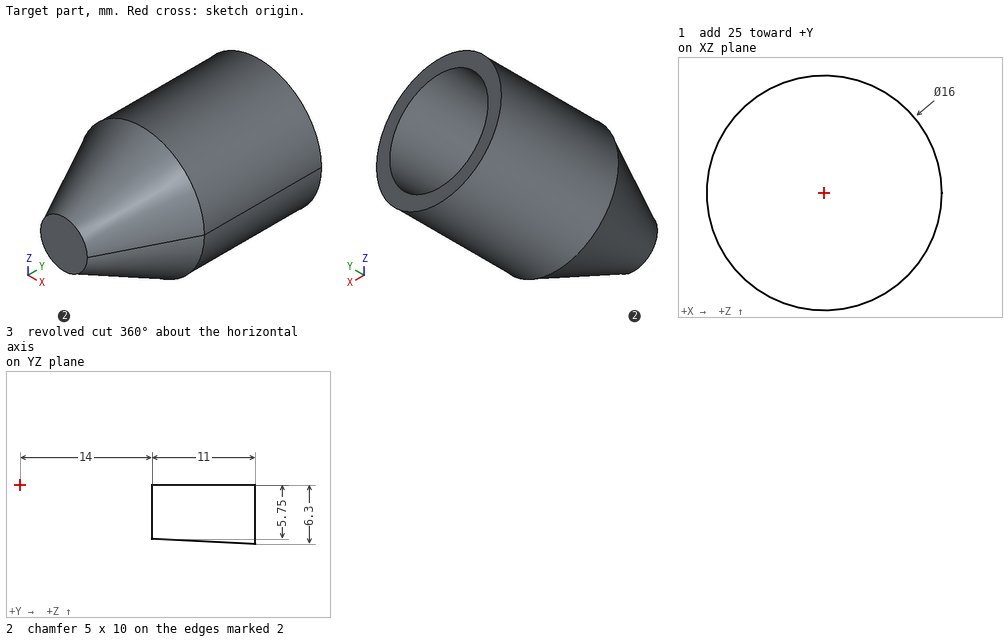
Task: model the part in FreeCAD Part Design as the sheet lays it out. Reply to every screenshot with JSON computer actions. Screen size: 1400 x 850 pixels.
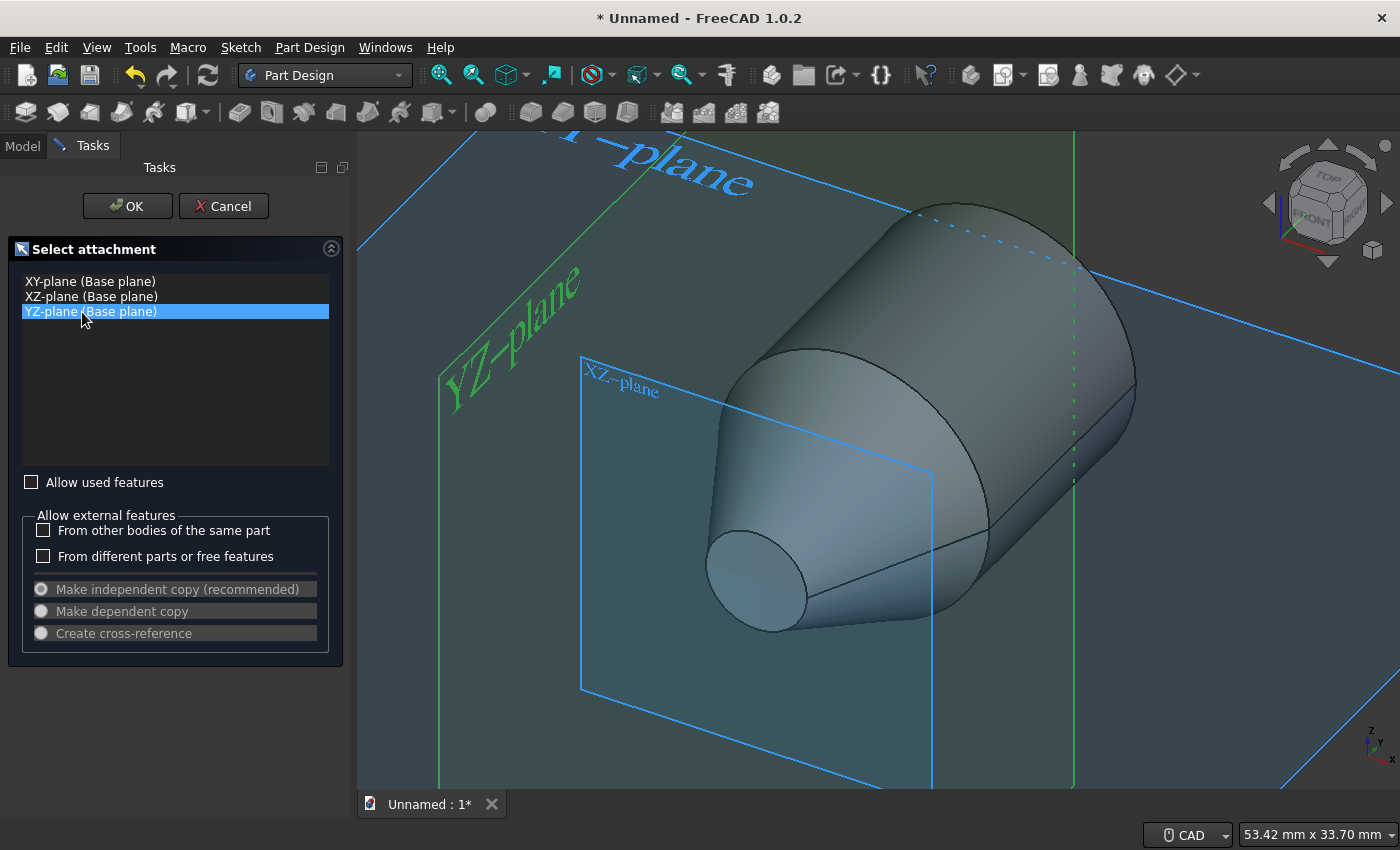
{"action": "left_click", "coordinate": [128, 206]}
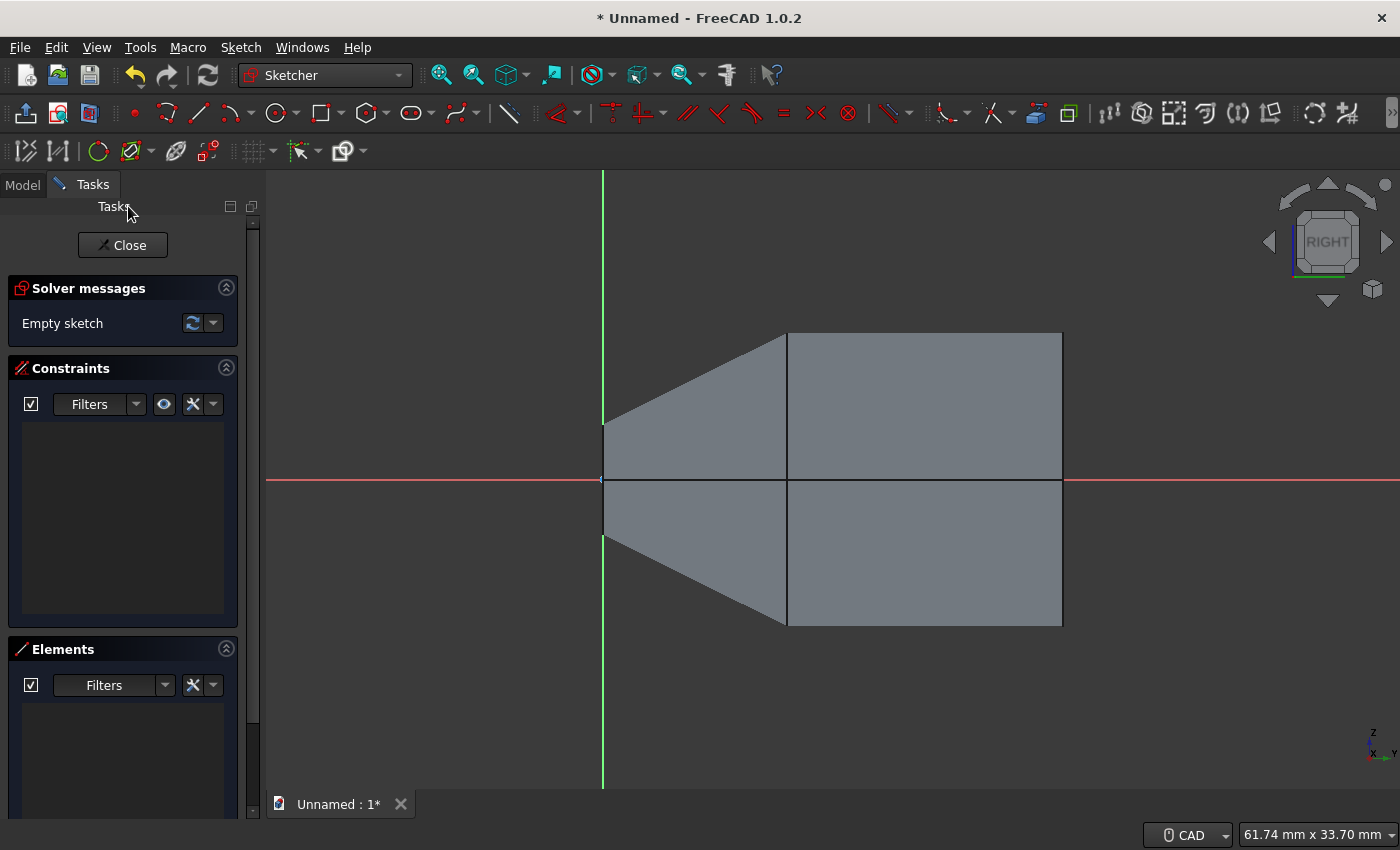
{"action": "left_click", "coordinate": [90, 114]}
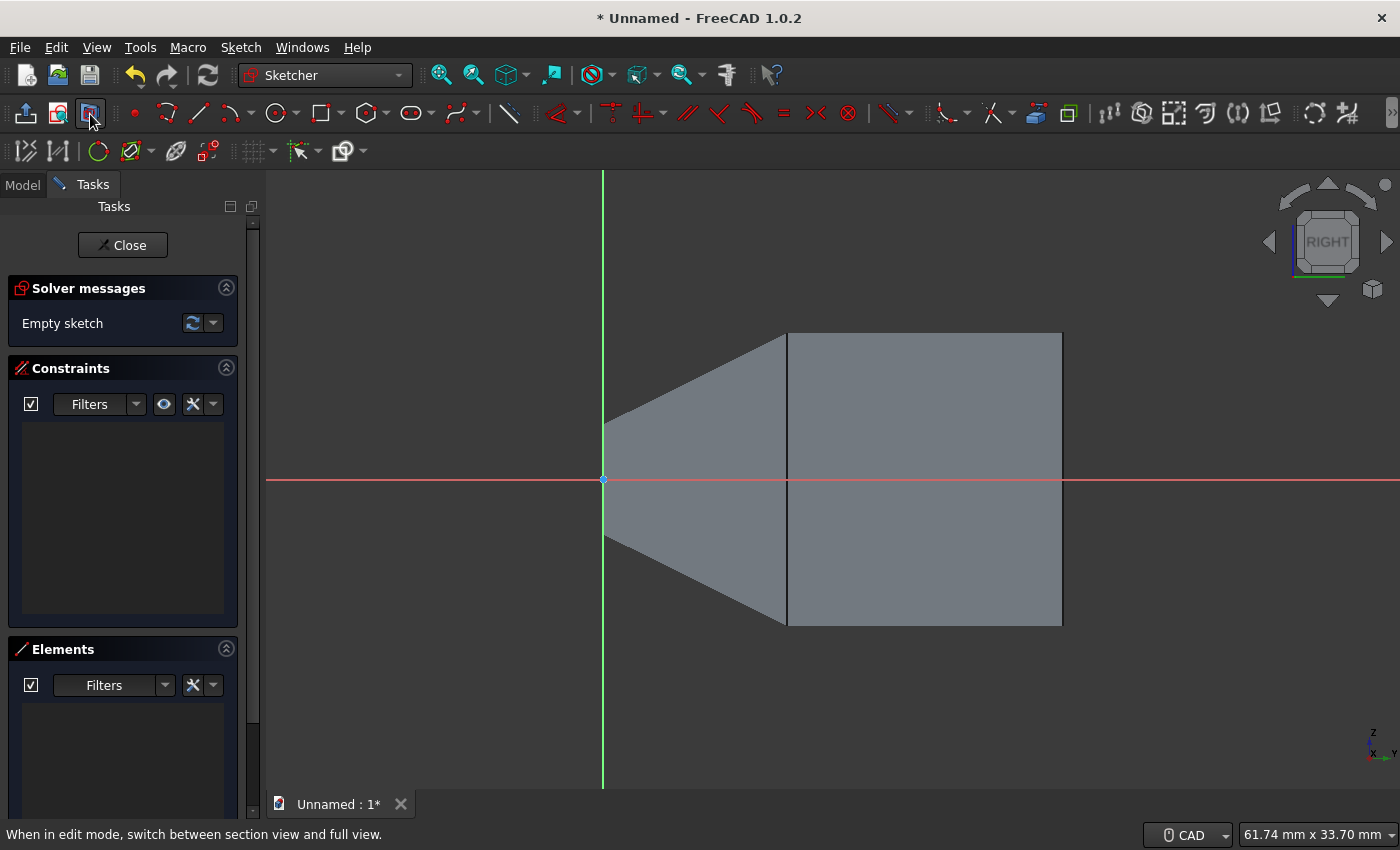
{"action": "scroll", "coordinate": [972, 655], "scroll_direction": "up", "scroll_amount": 2}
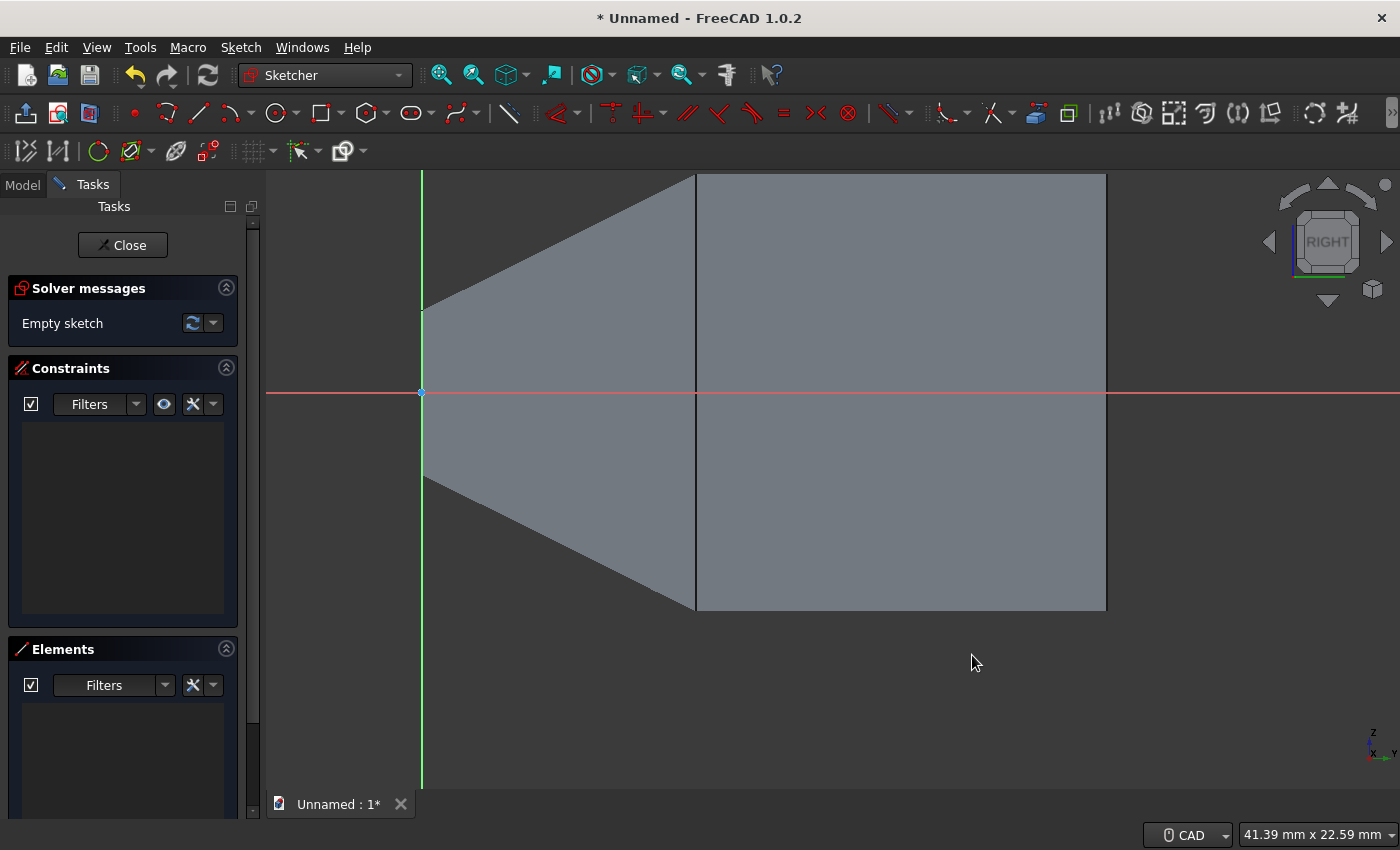
{"action": "left_click", "coordinate": [168, 114]}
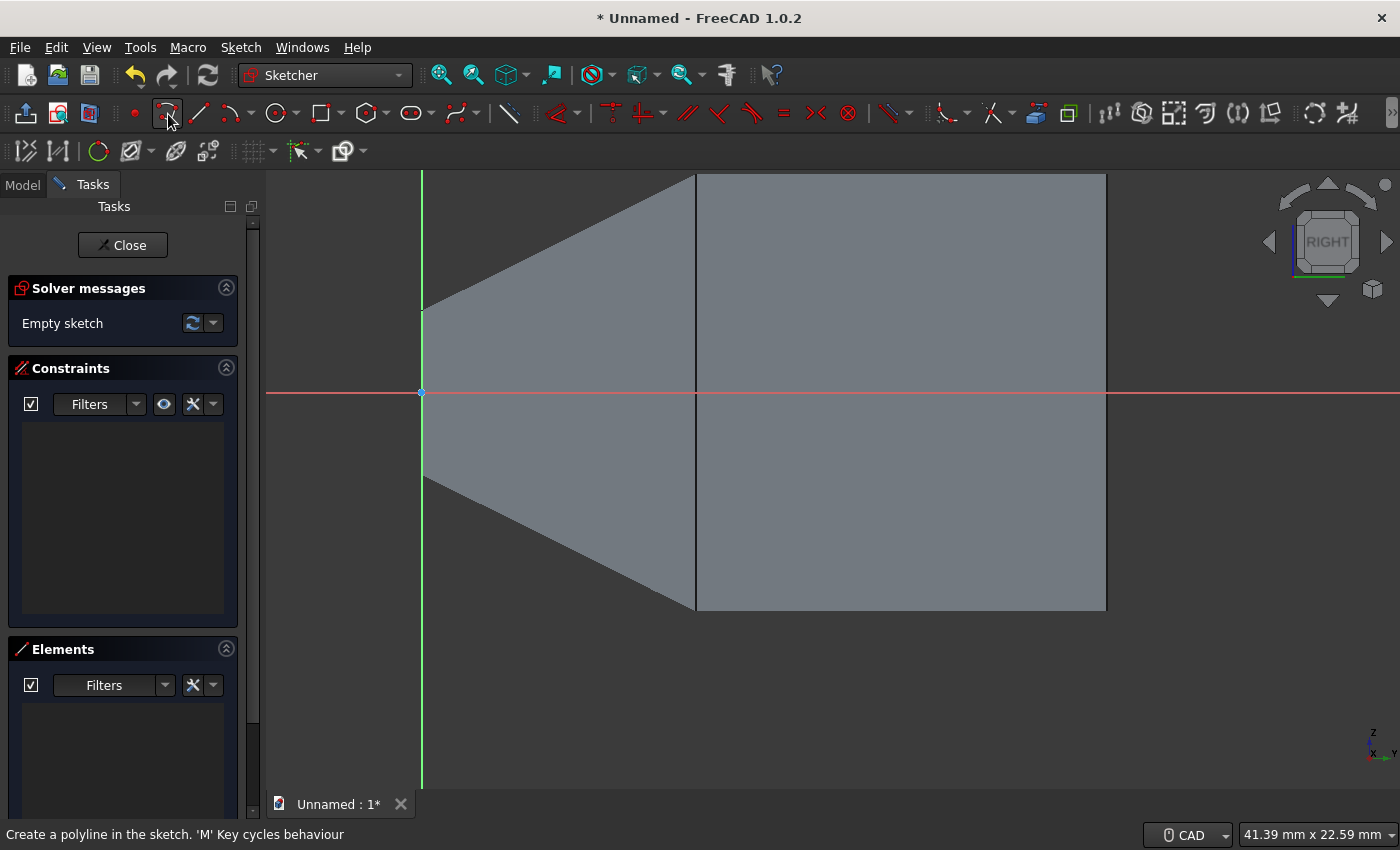
{"action": "left_click", "coordinate": [805, 393]}
{"action": "left_click", "coordinate": [805, 550]}
{"action": "left_click", "coordinate": [1107, 565]}
{"action": "left_click", "coordinate": [1107, 402]}
{"action": "left_click", "coordinate": [805, 393]}
{"action": "key", "text": "Escape"}
{"action": "key", "text": "Escape"}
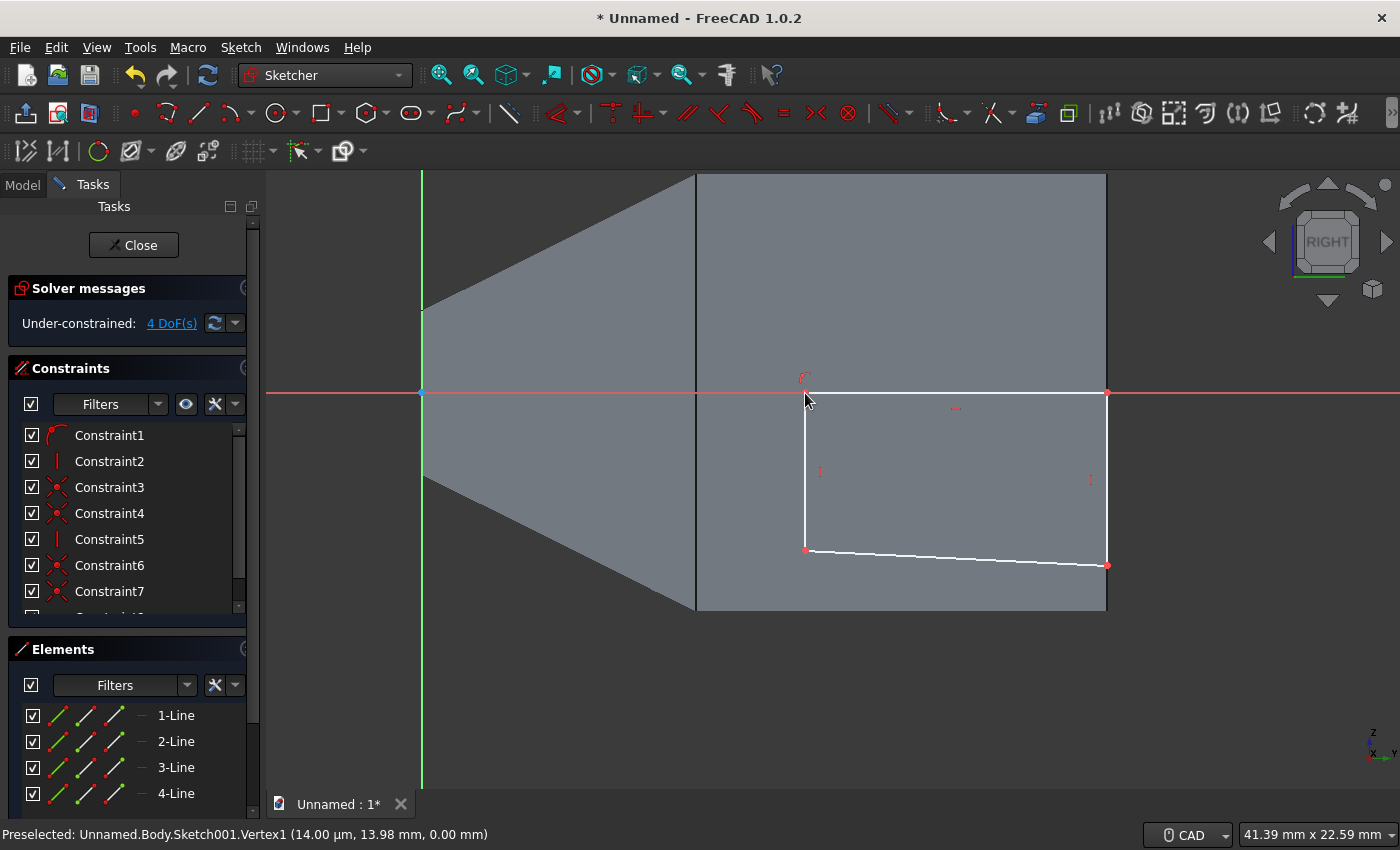
{"action": "left_click", "coordinate": [556, 114]}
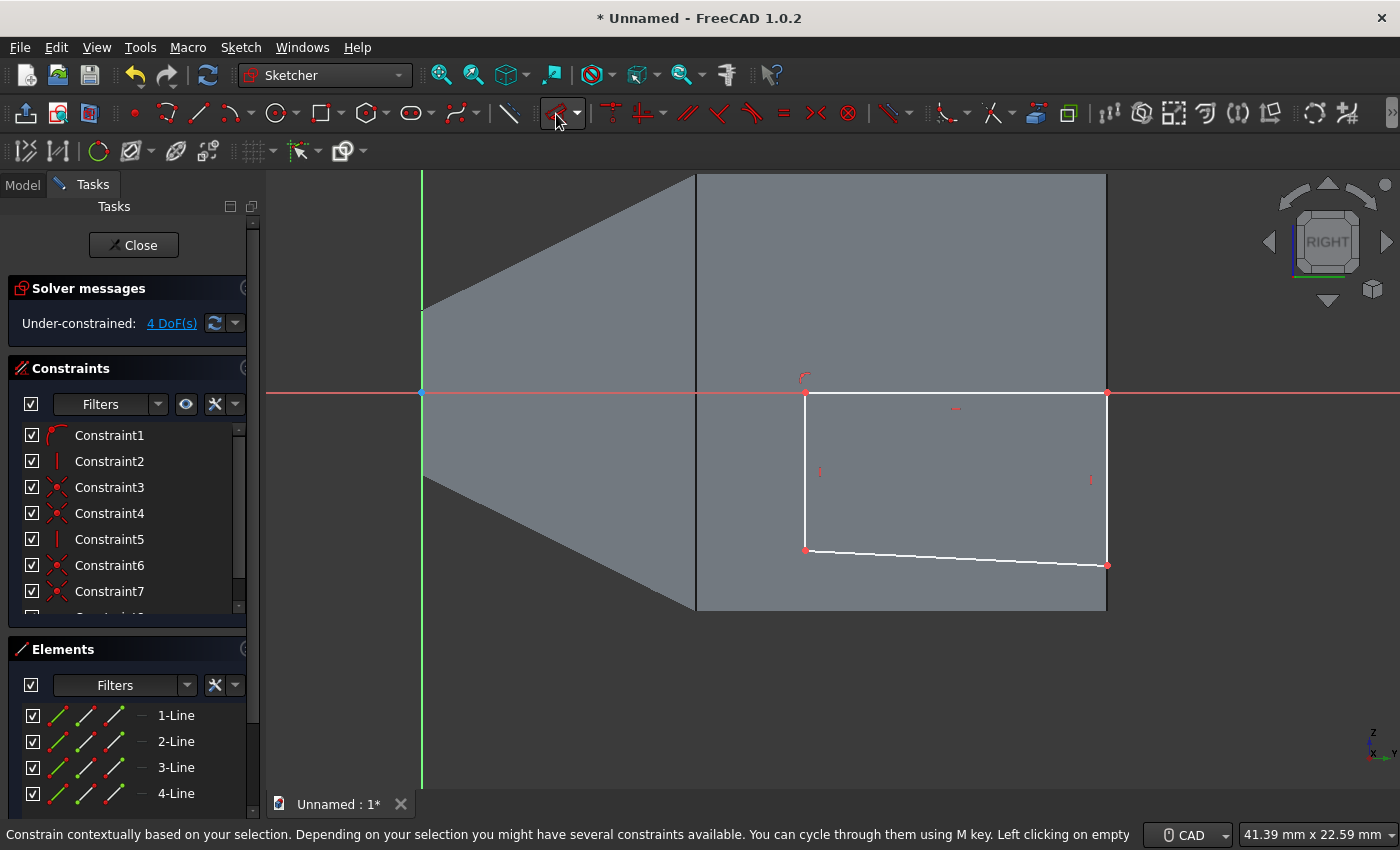
{"action": "left_click", "coordinate": [1016, 393]}
{"action": "left_click", "coordinate": [956, 359]}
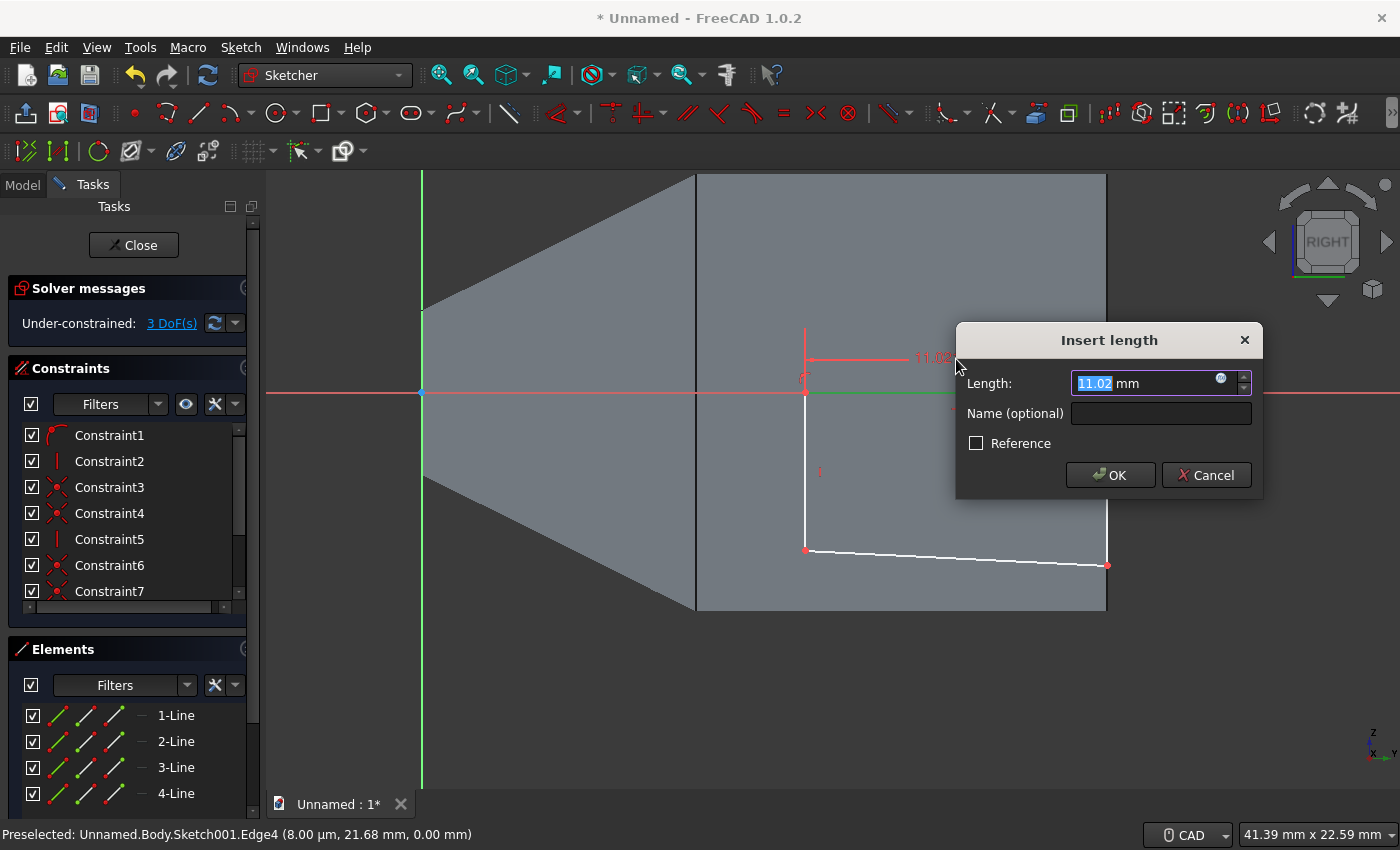
{"action": "type", "text": "11"}
{"action": "key", "text": "Return"}